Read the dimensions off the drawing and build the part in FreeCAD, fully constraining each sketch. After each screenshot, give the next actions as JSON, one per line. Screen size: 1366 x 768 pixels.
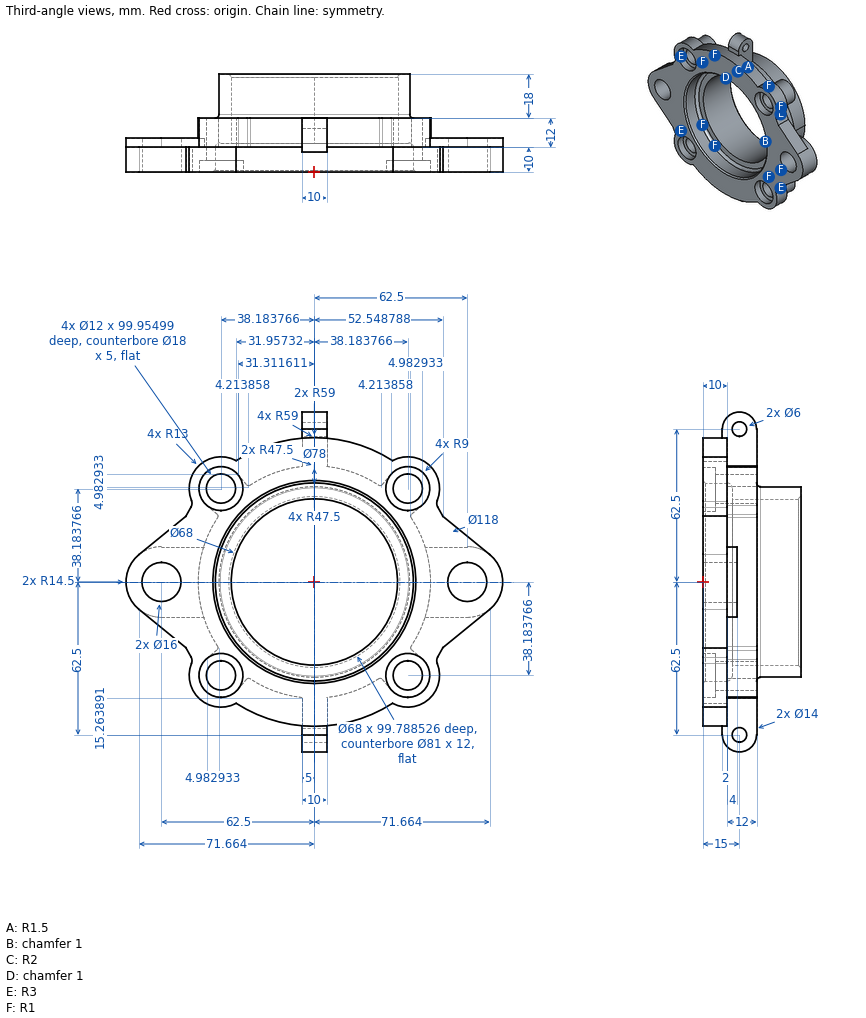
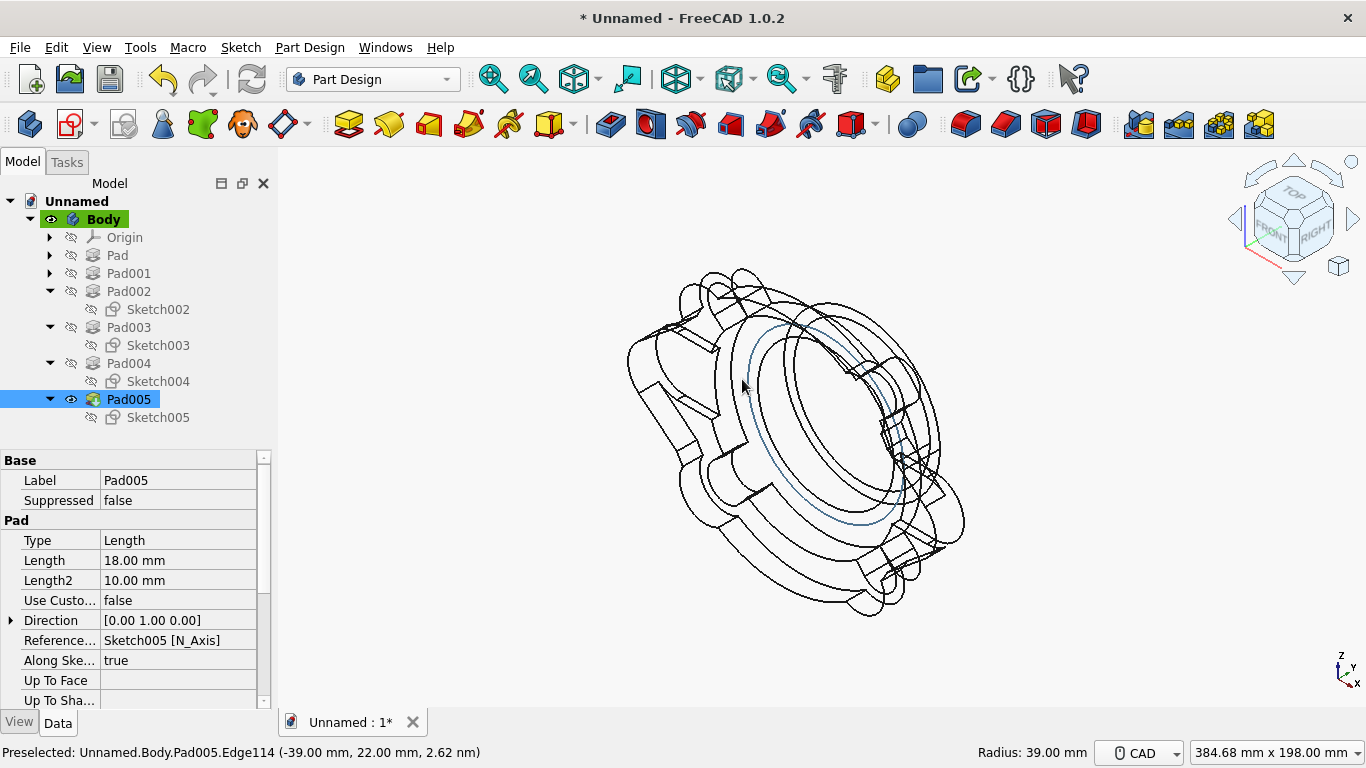
{"action": "key", "text": "v 1"}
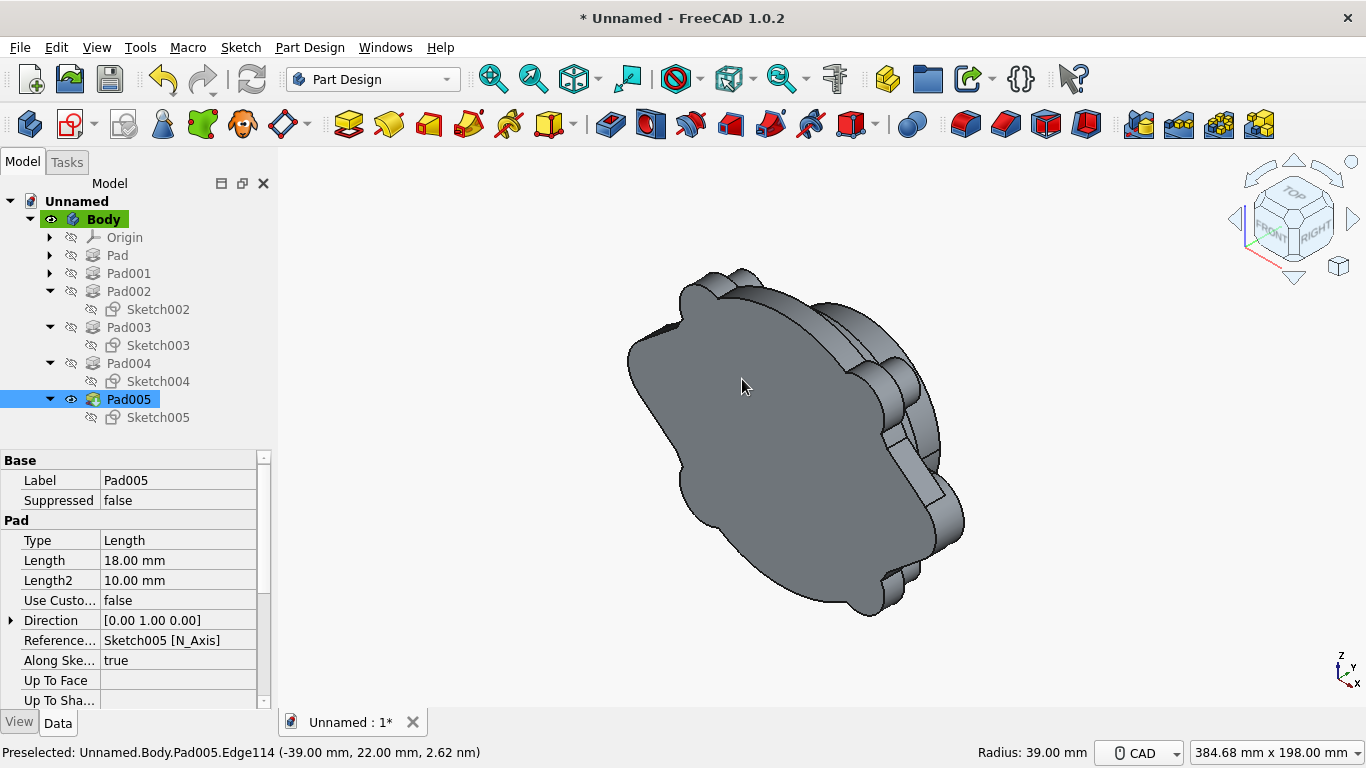
{"action": "left_click", "coordinate": [966, 124]}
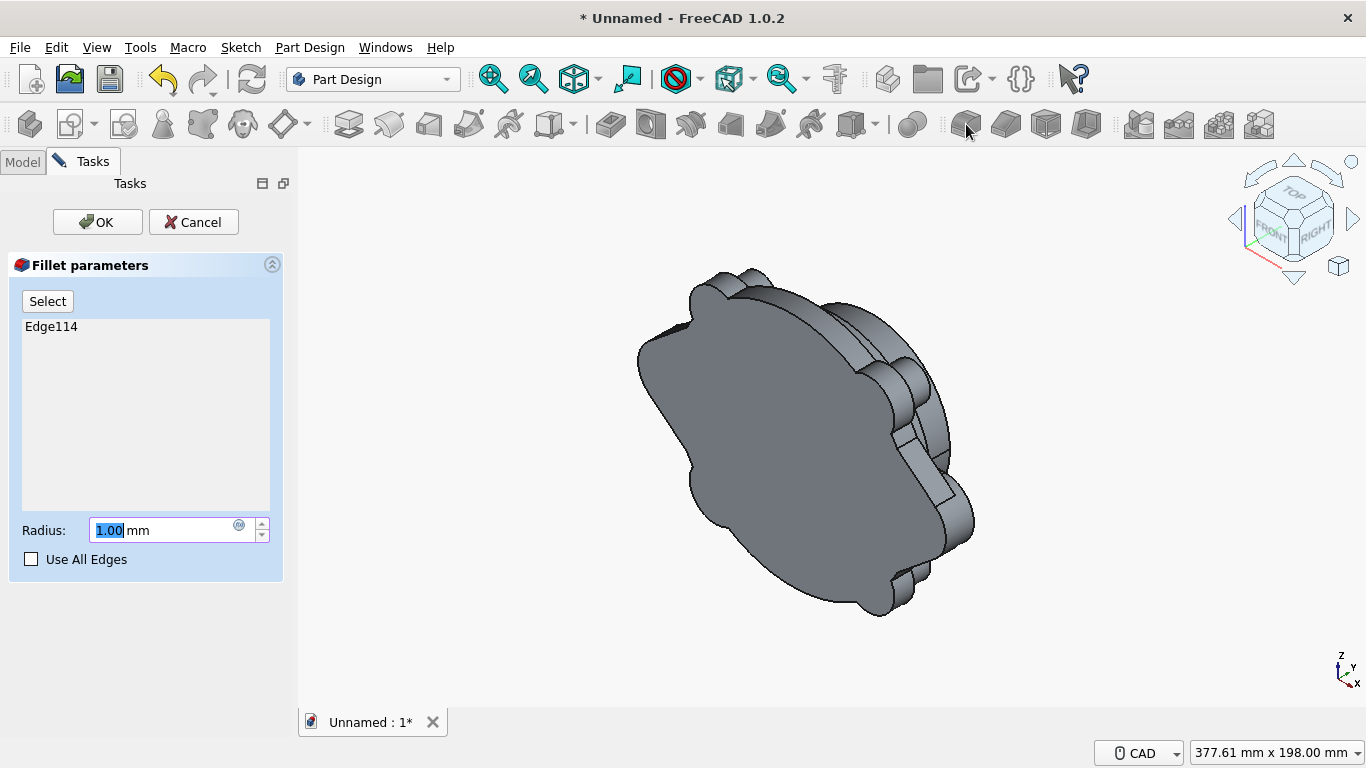
{"action": "type", "text": "1.5"}
{"action": "key", "text": "Tab"}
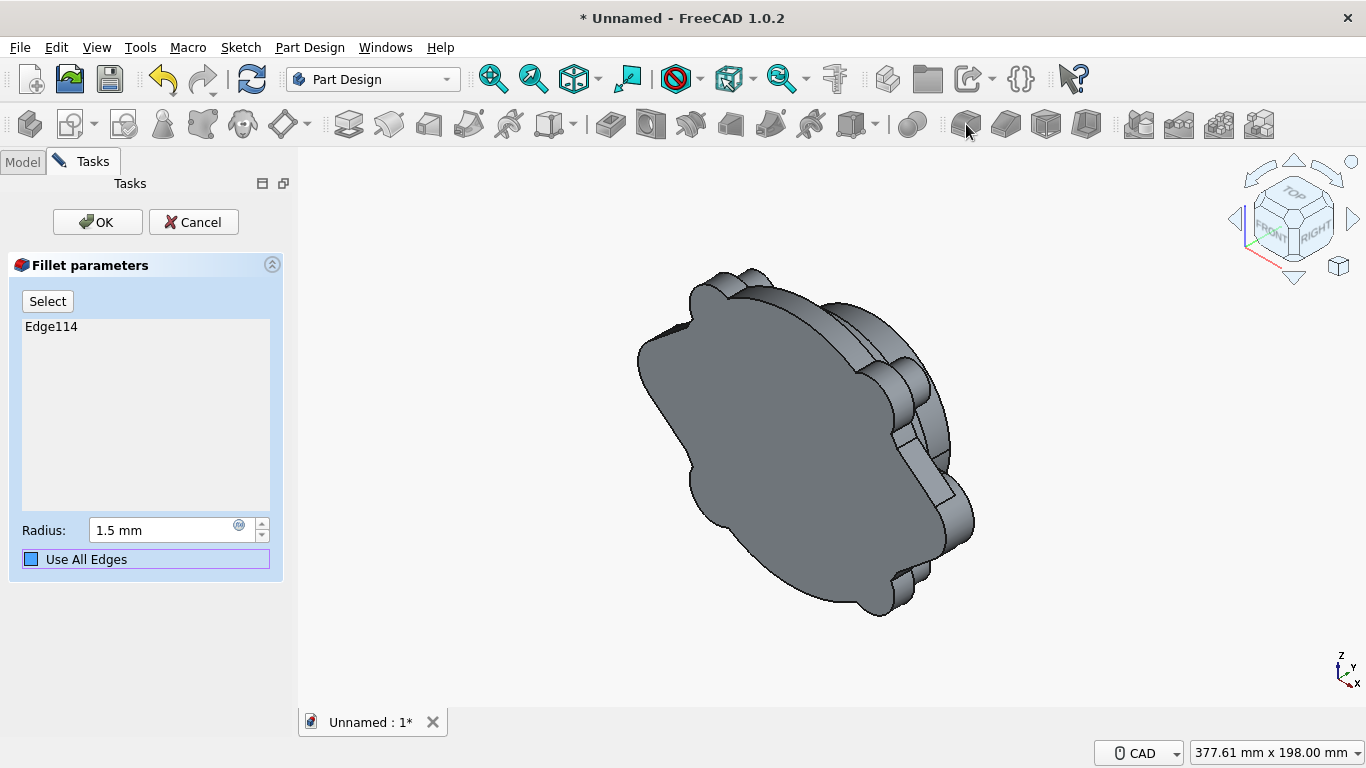
{"action": "left_click", "coordinate": [98, 222]}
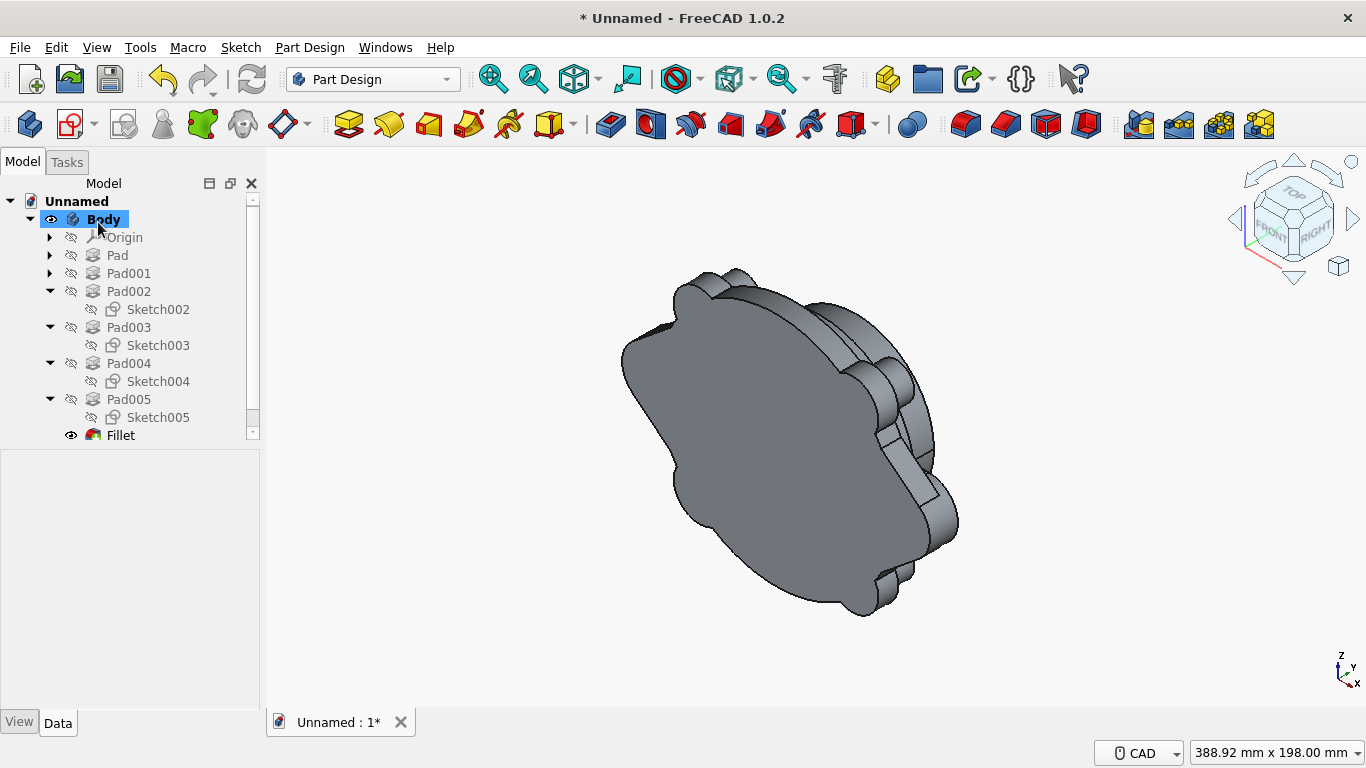
{"action": "key", "text": "2"}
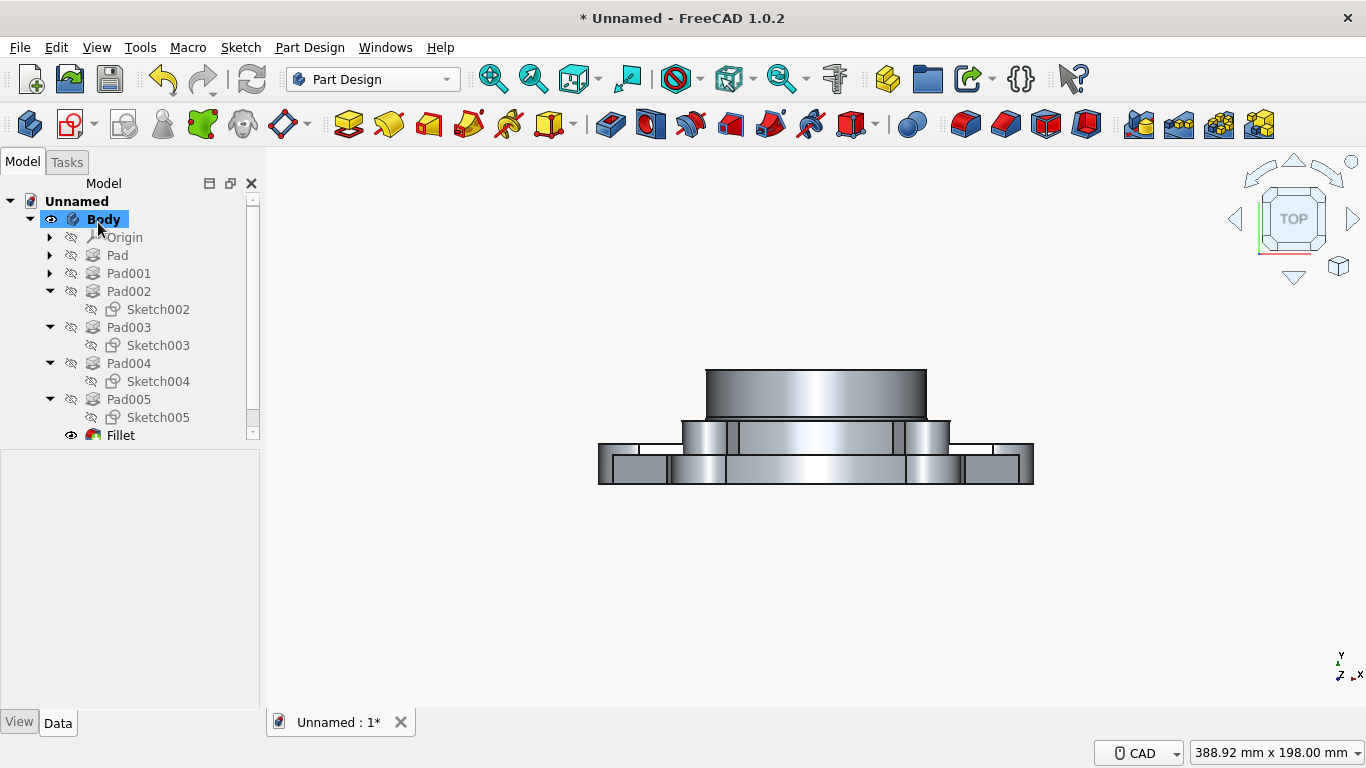
{"action": "left_click", "coordinate": [494, 80]}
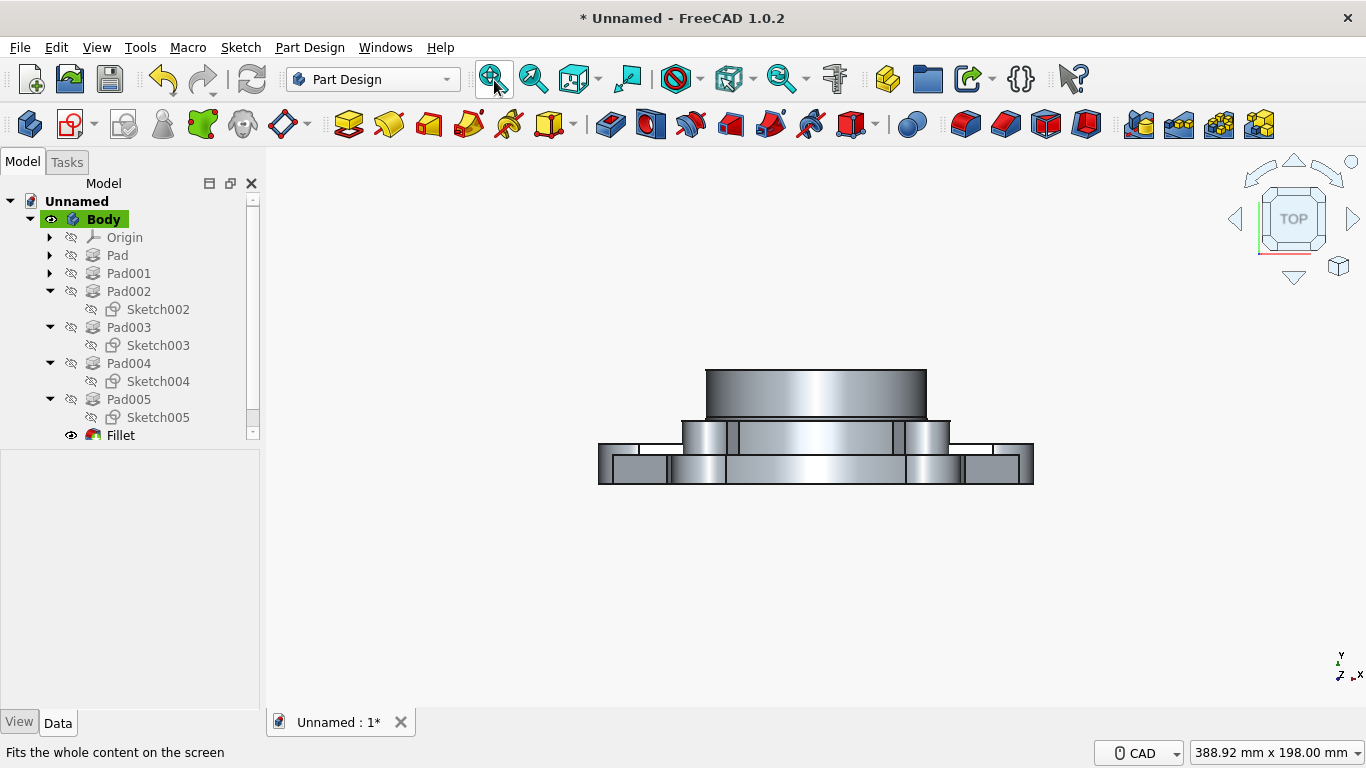
{"action": "key", "text": "0"}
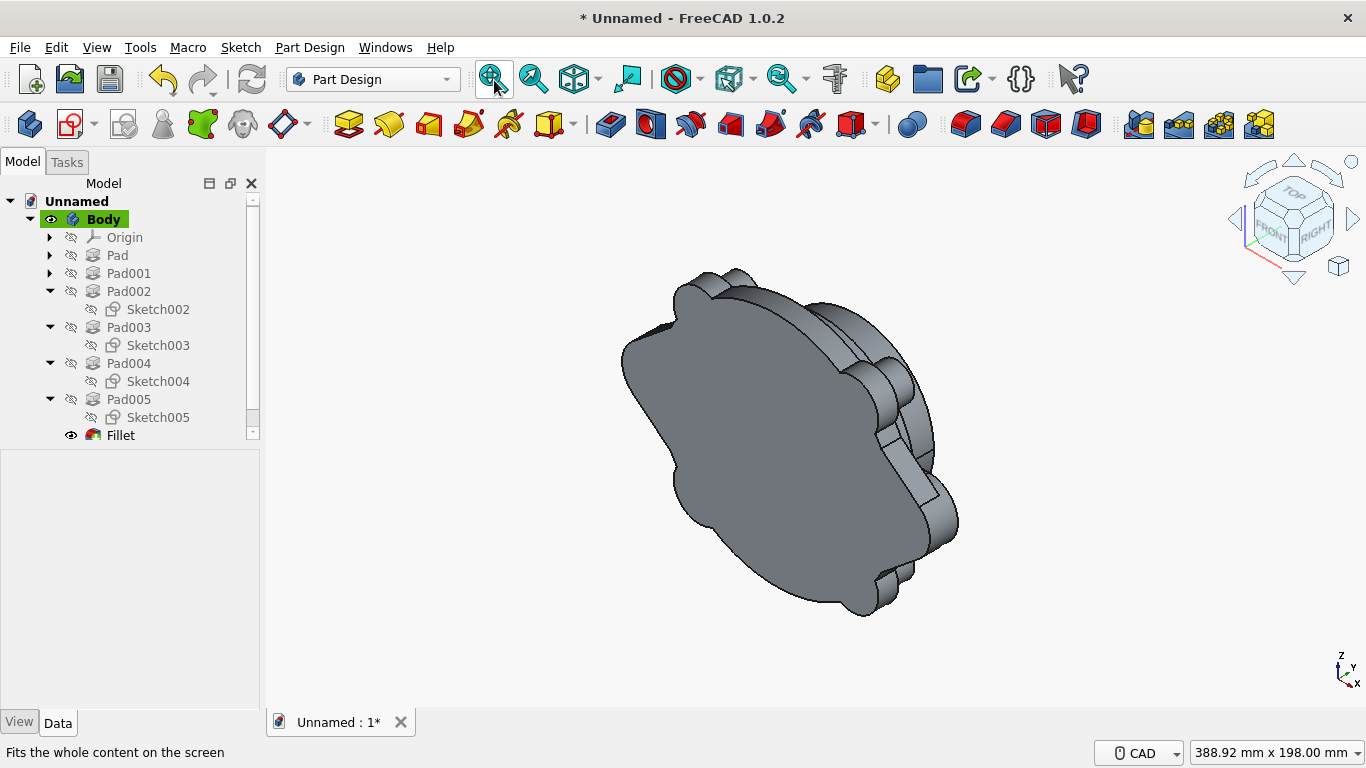
{"action": "key", "text": "1"}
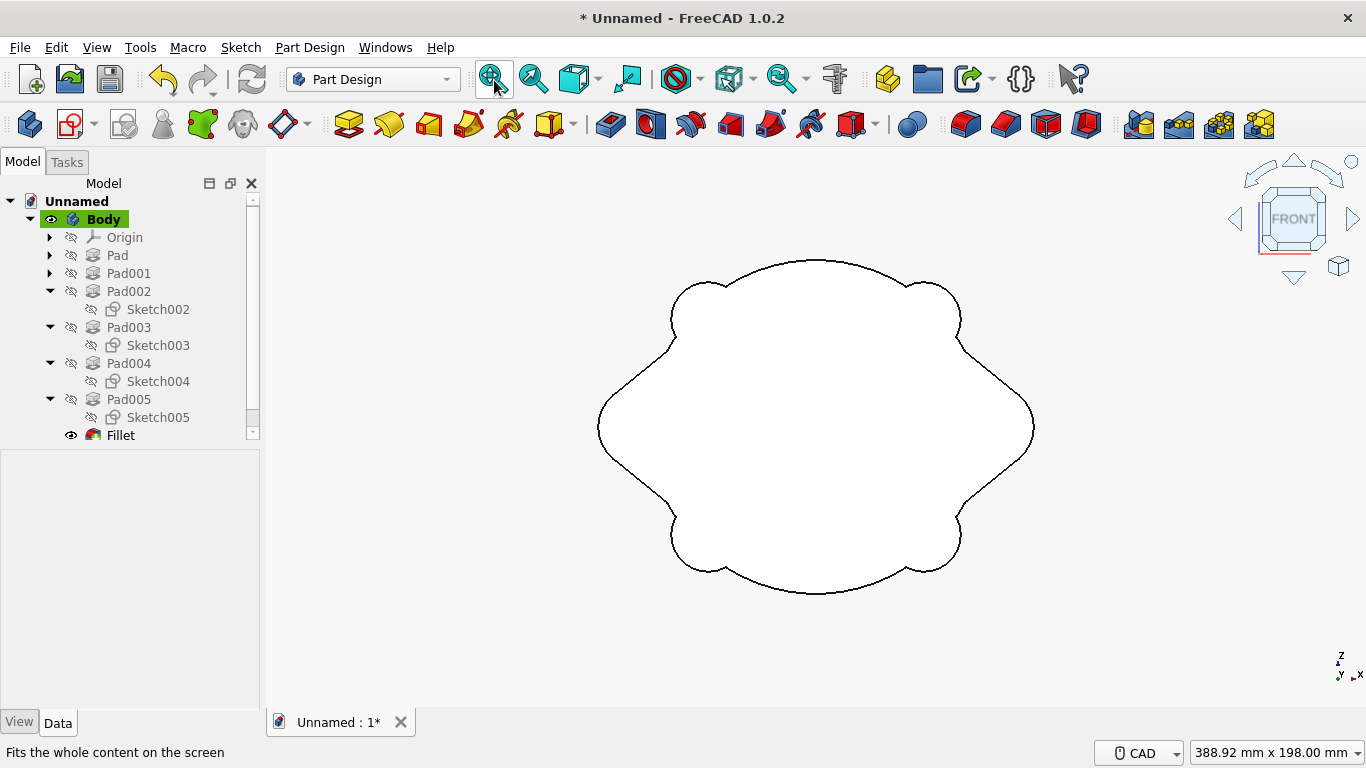
{"action": "key", "text": "3"}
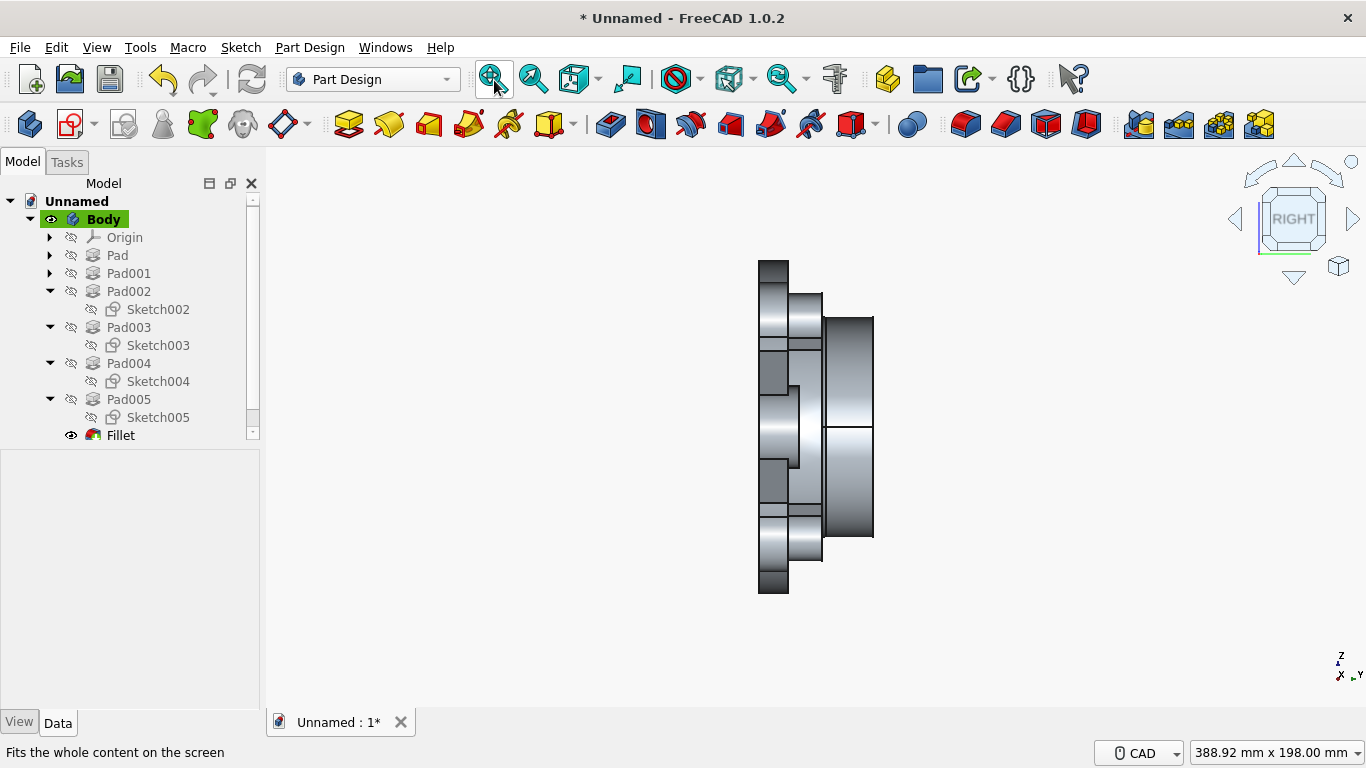
{"action": "key", "text": "5"}